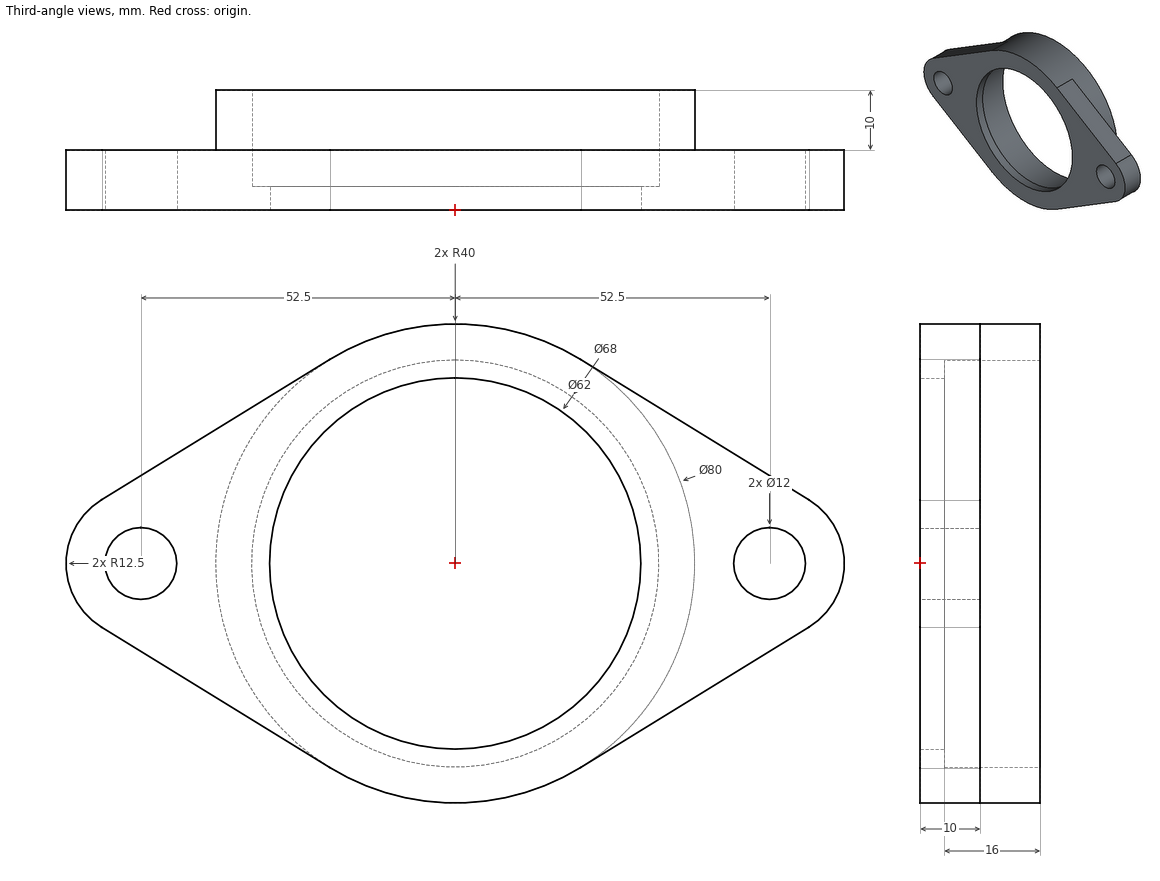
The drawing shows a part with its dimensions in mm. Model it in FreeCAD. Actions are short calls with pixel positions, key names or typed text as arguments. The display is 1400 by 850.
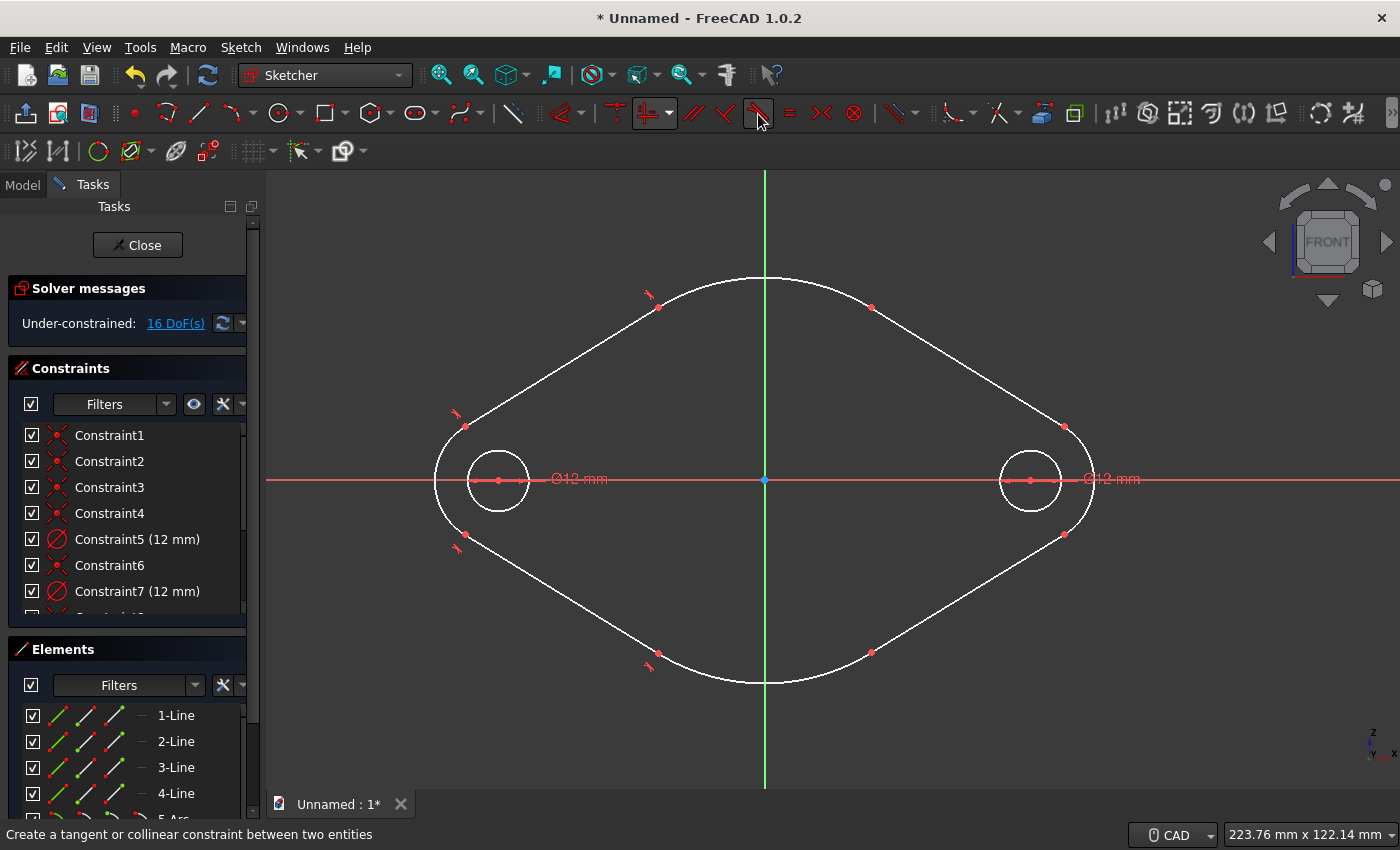
click(929, 344)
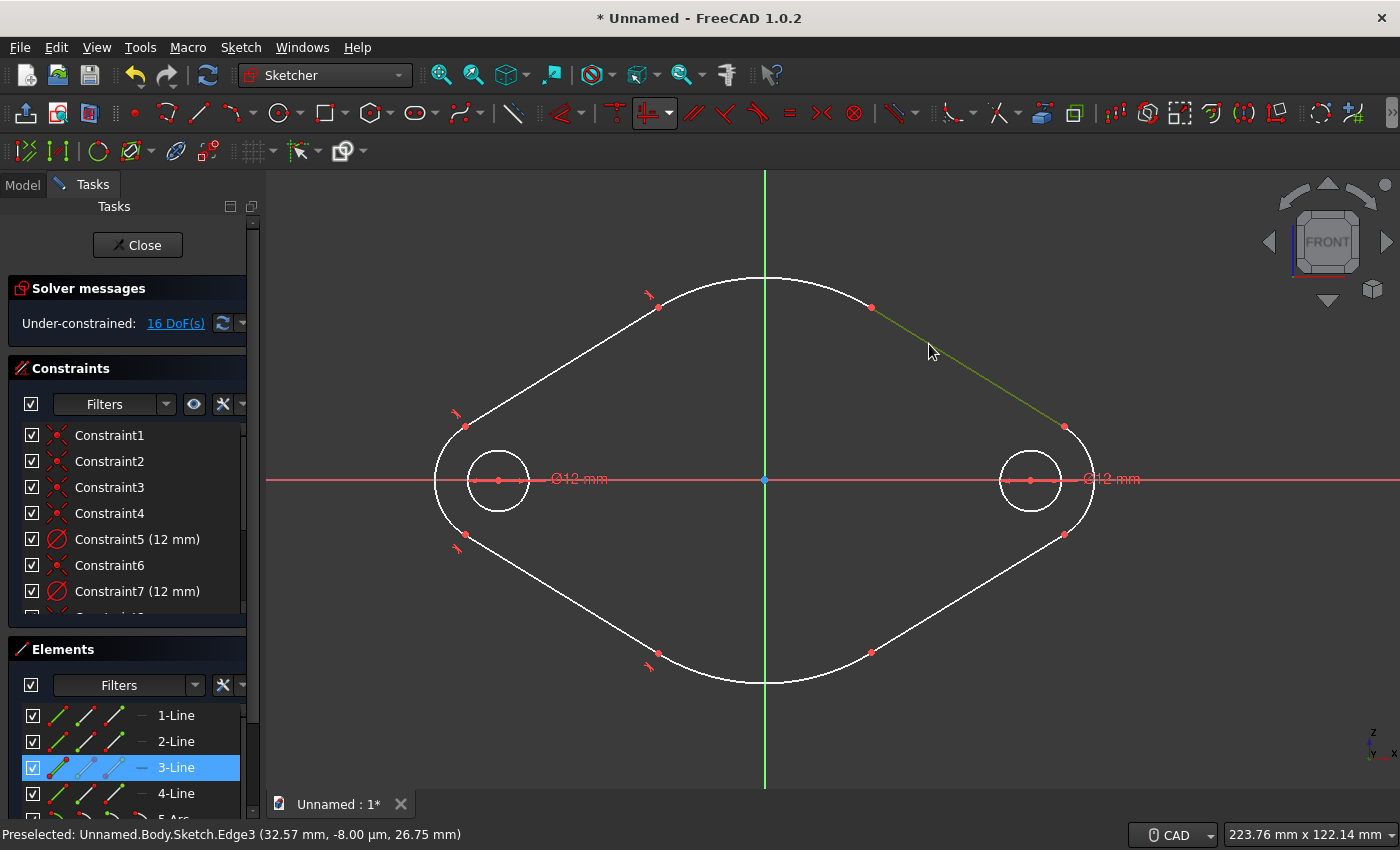
click(809, 283)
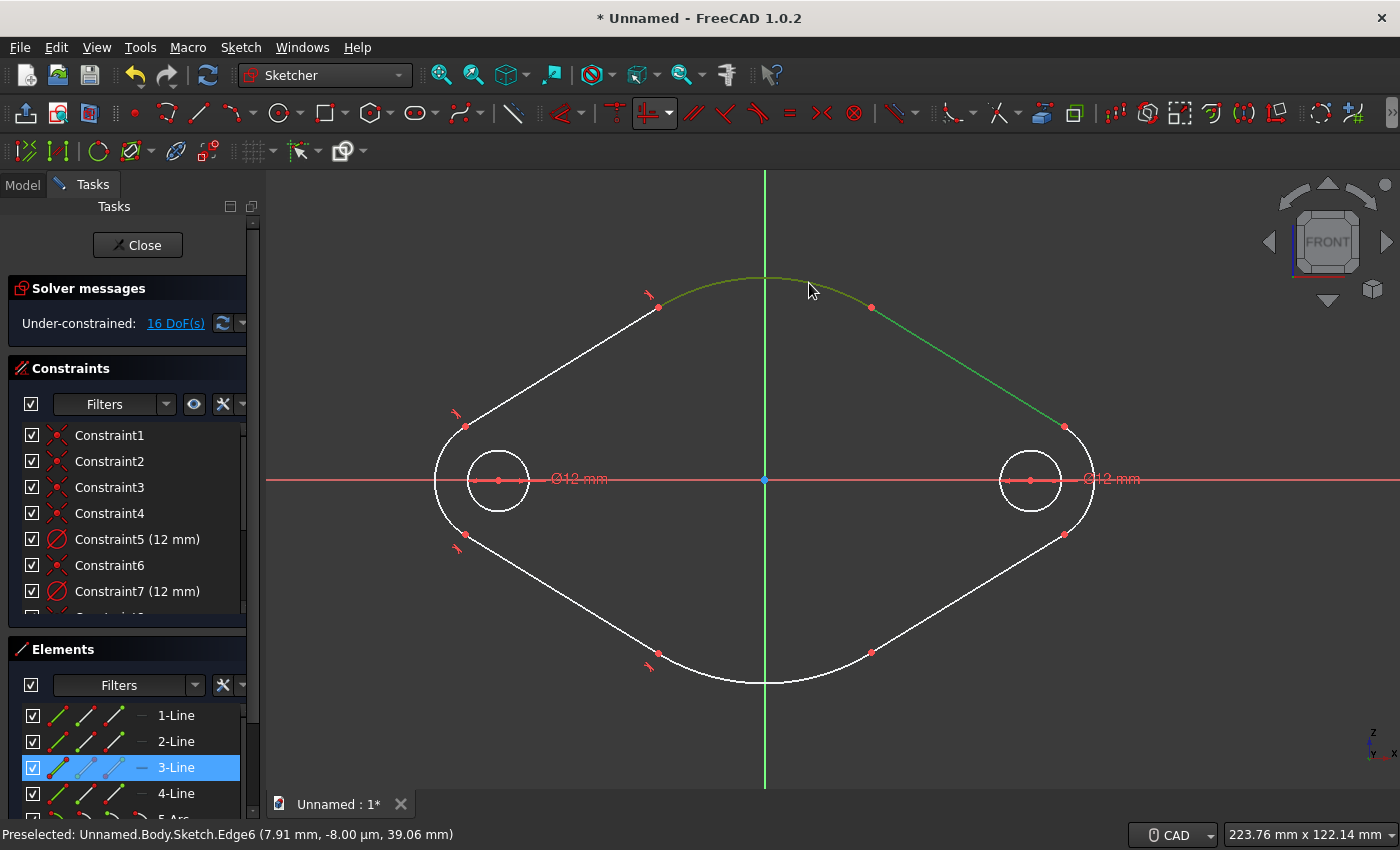
click(758, 114)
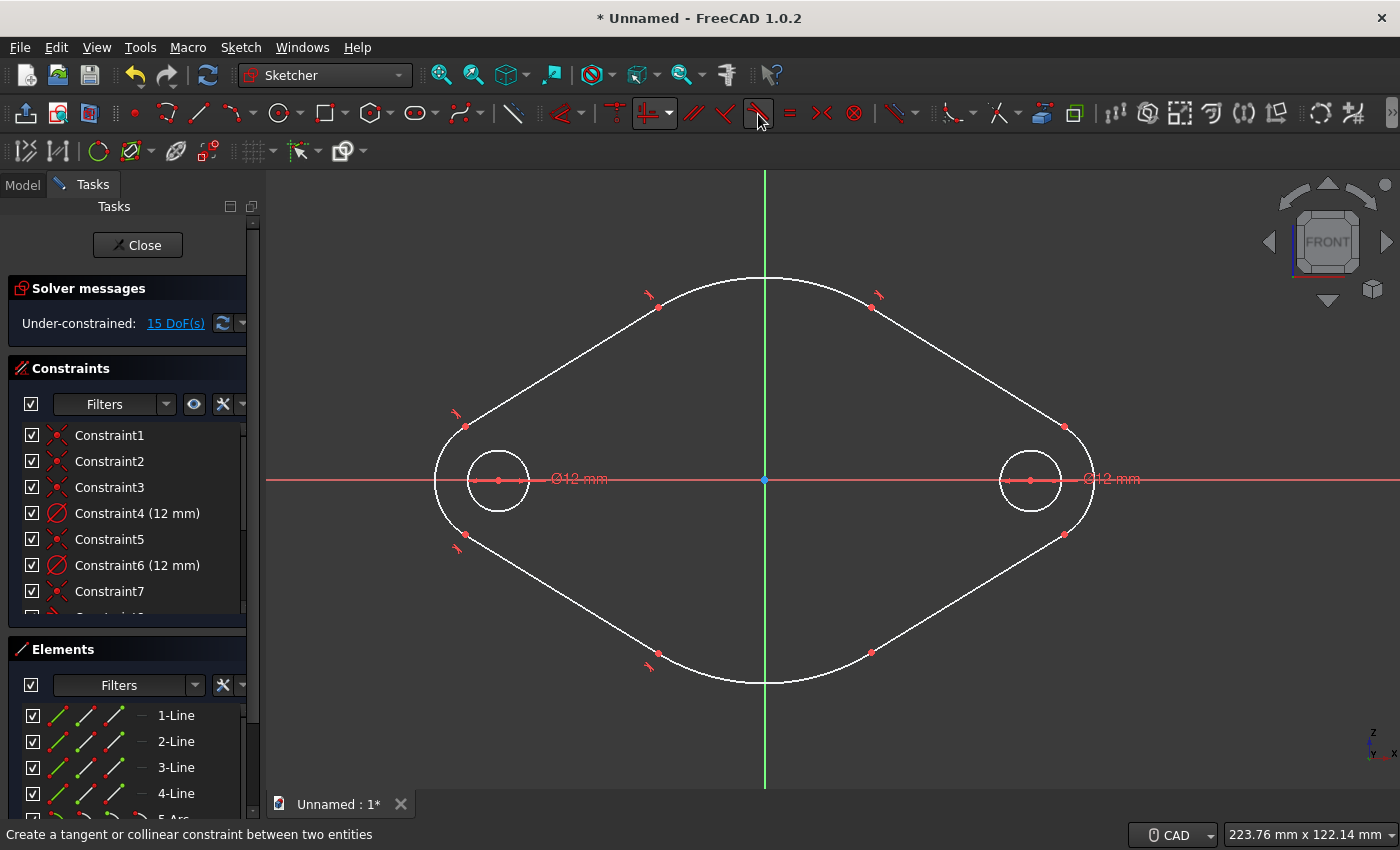
click(929, 344)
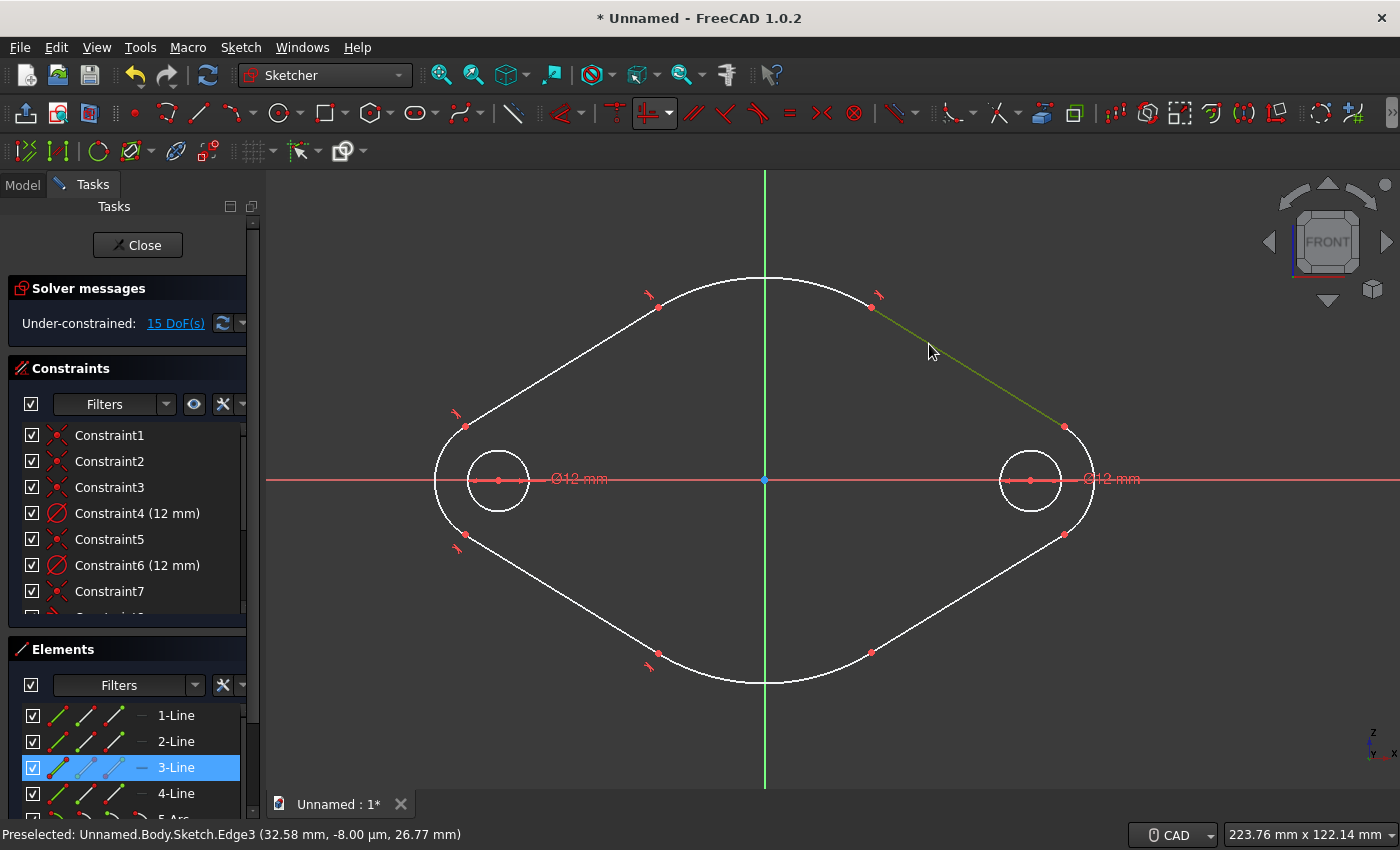
click(1089, 506)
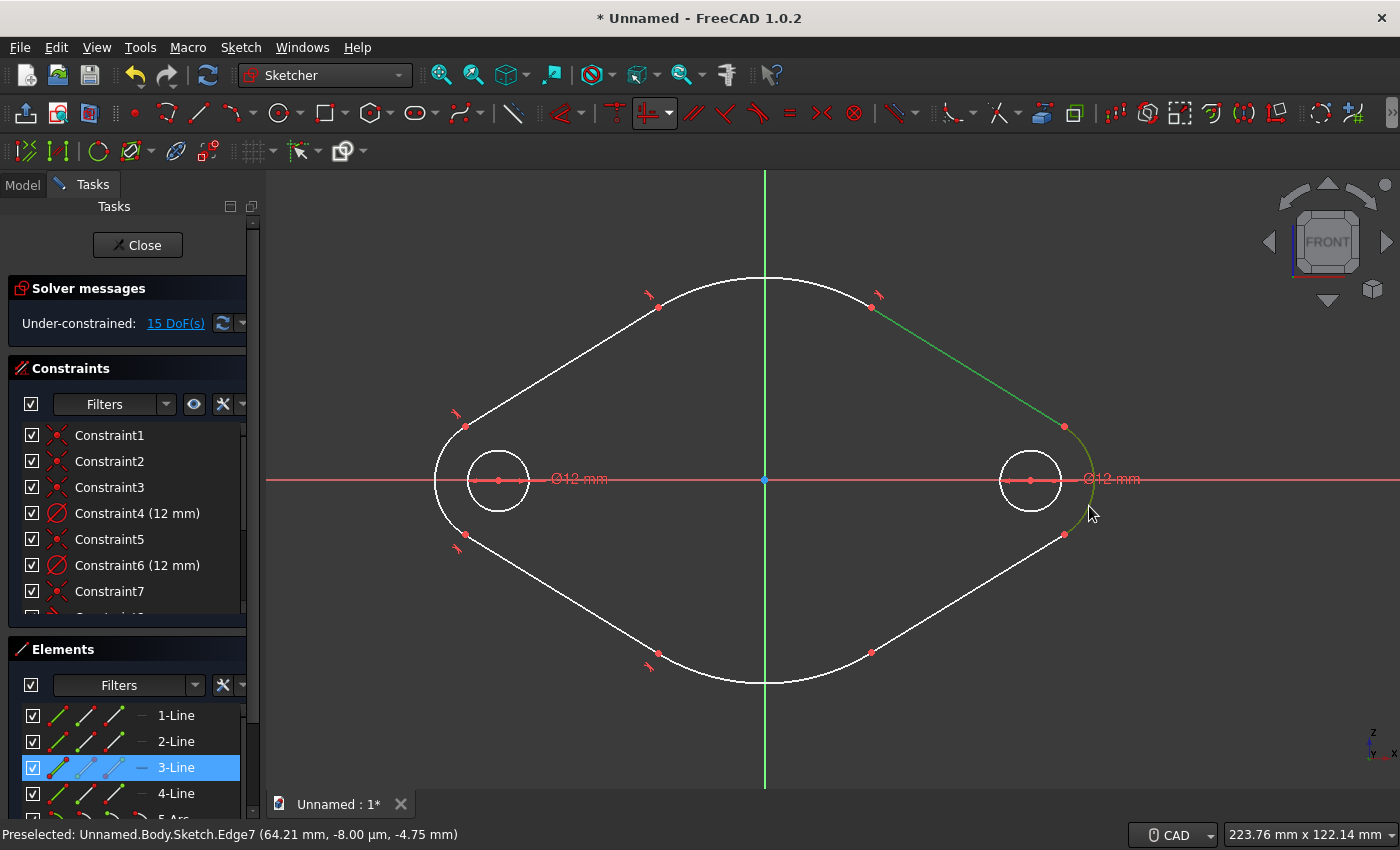
click(758, 114)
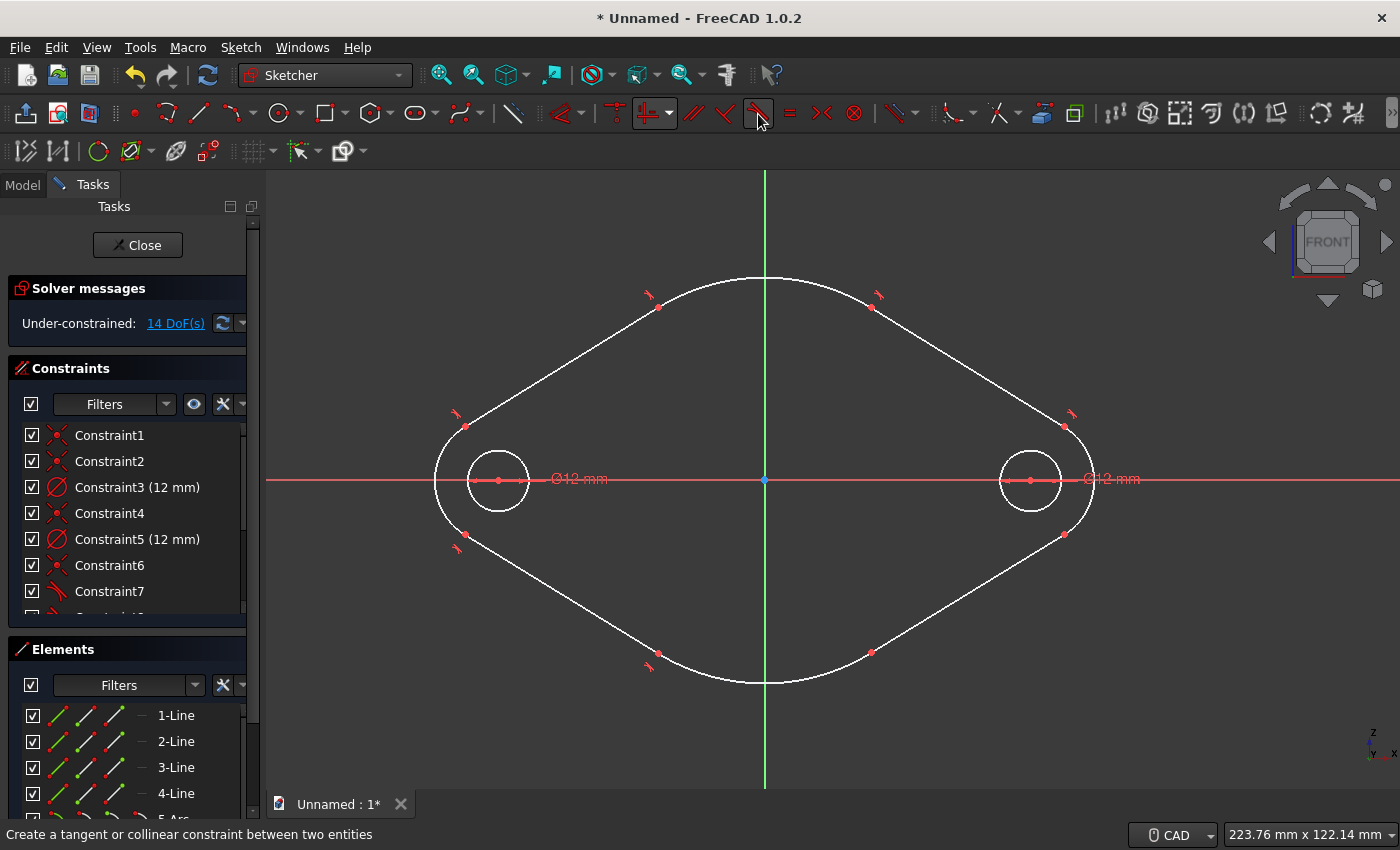
click(1006, 570)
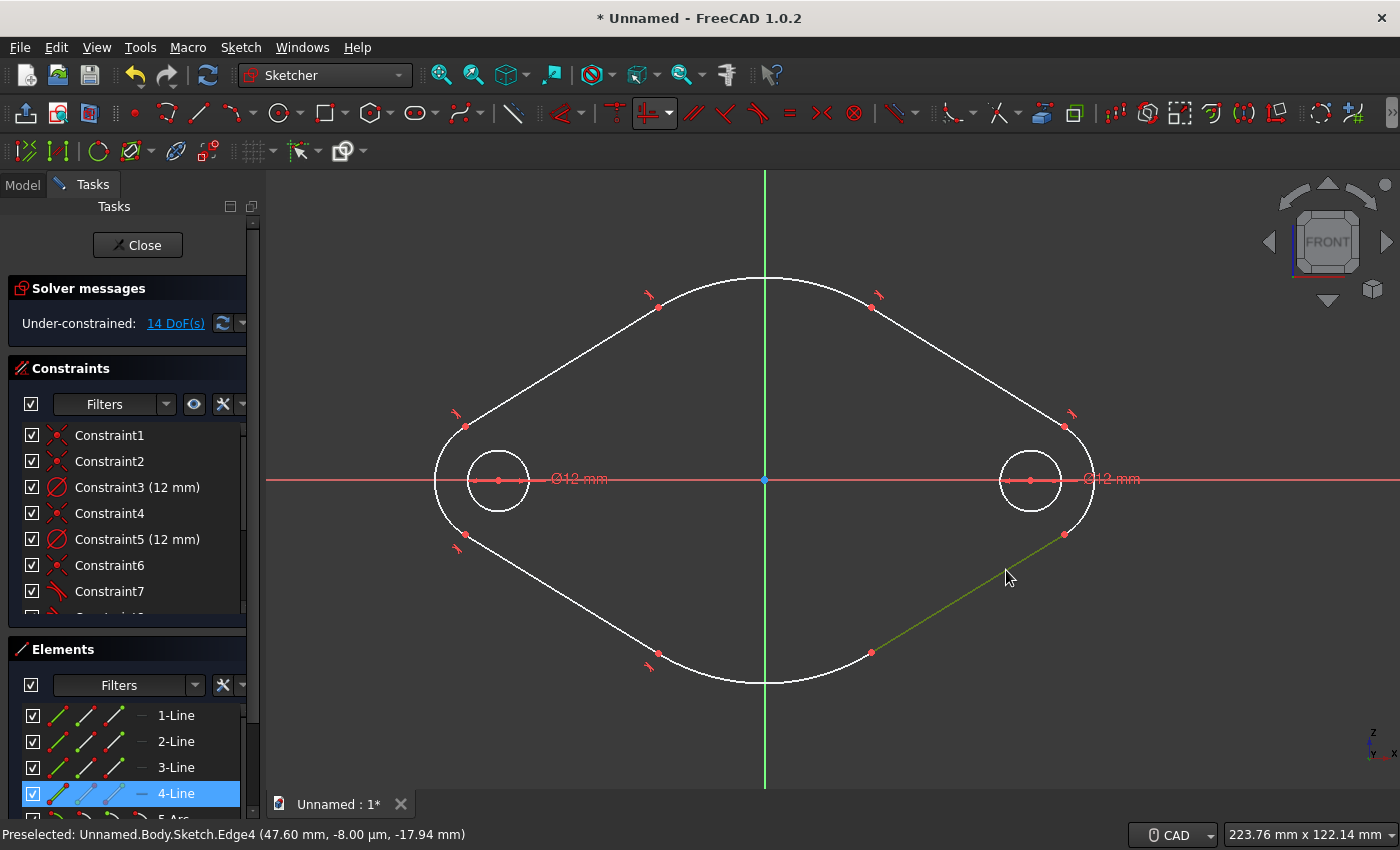
click(1089, 506)